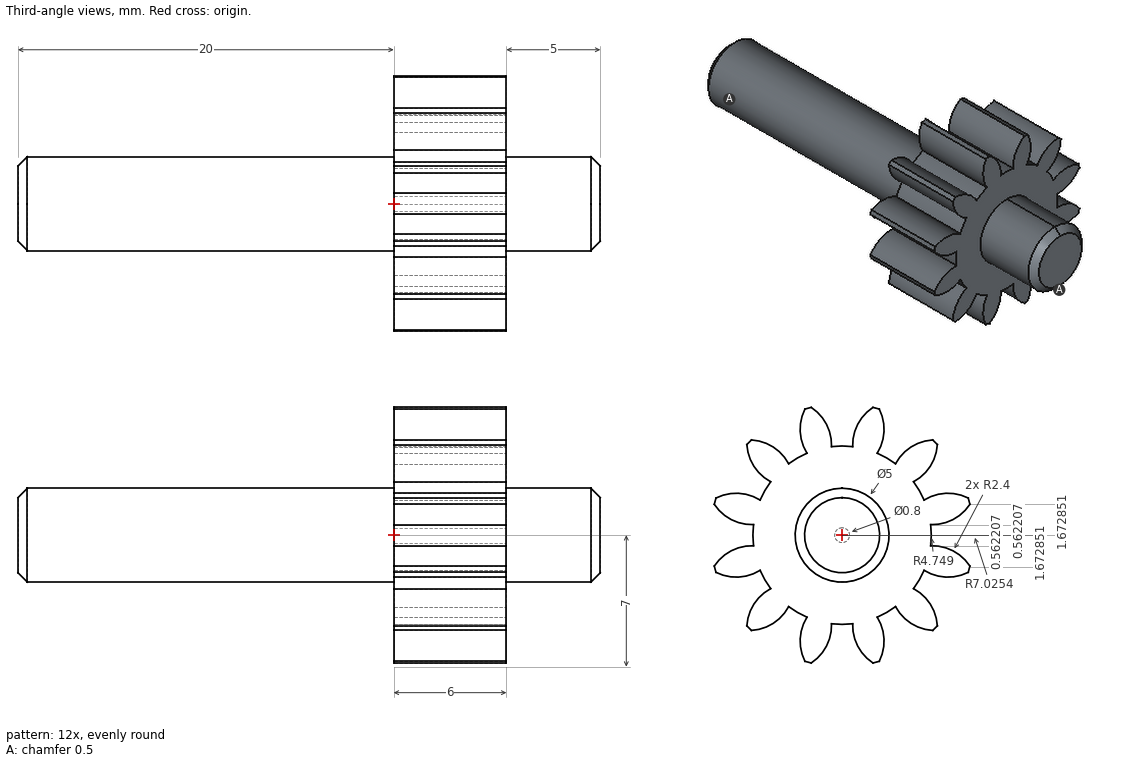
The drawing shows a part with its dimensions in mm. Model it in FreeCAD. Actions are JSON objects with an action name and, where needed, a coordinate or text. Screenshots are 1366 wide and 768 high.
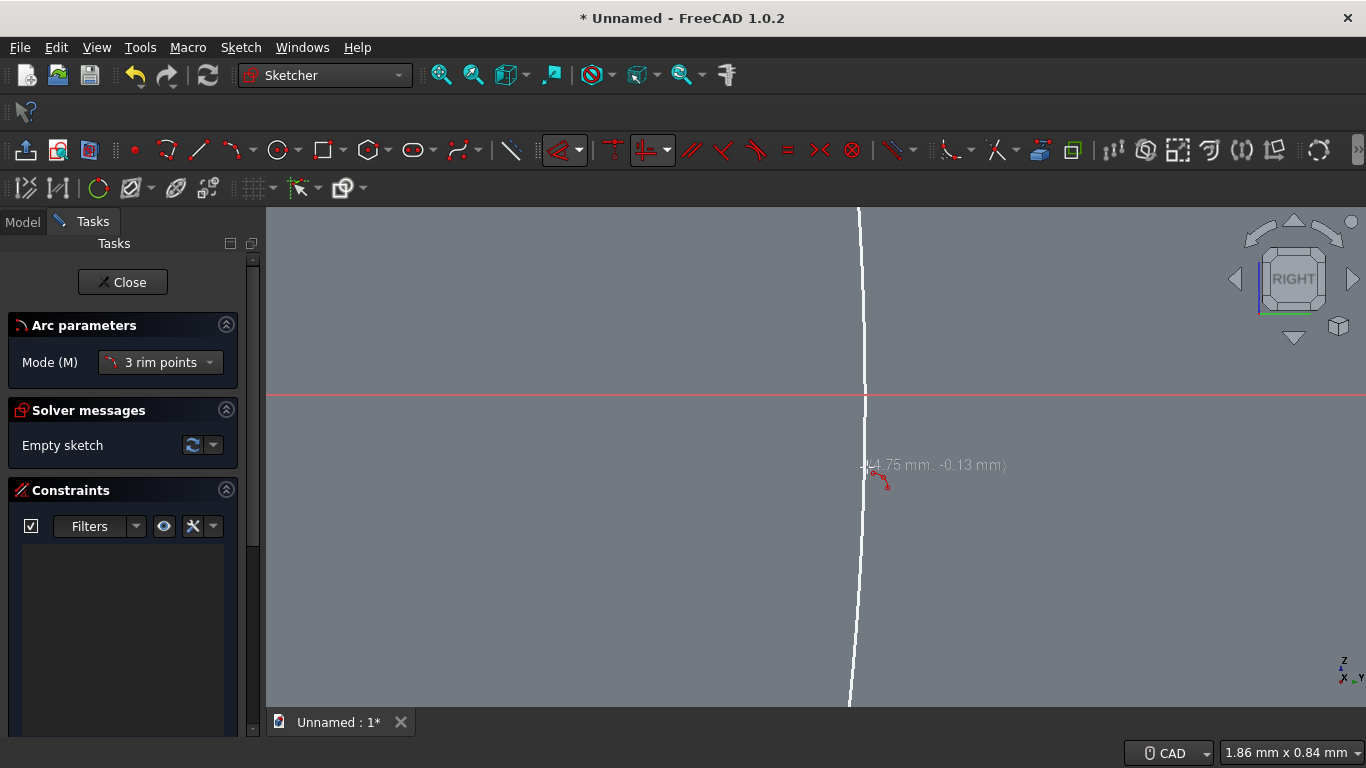
{"action": "left_click", "coordinate": [864, 461]}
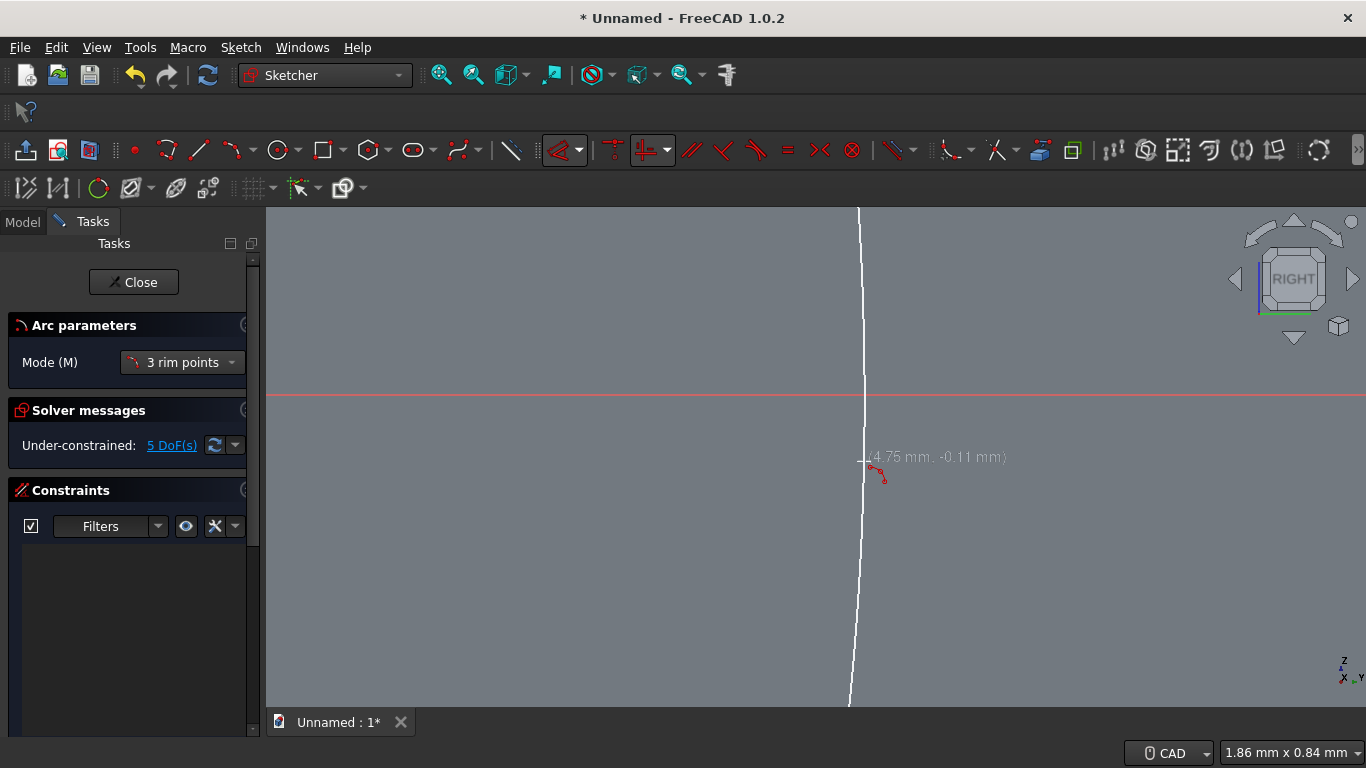
{"action": "scroll", "coordinate": [869, 469], "scroll_direction": "down", "scroll_amount": 9}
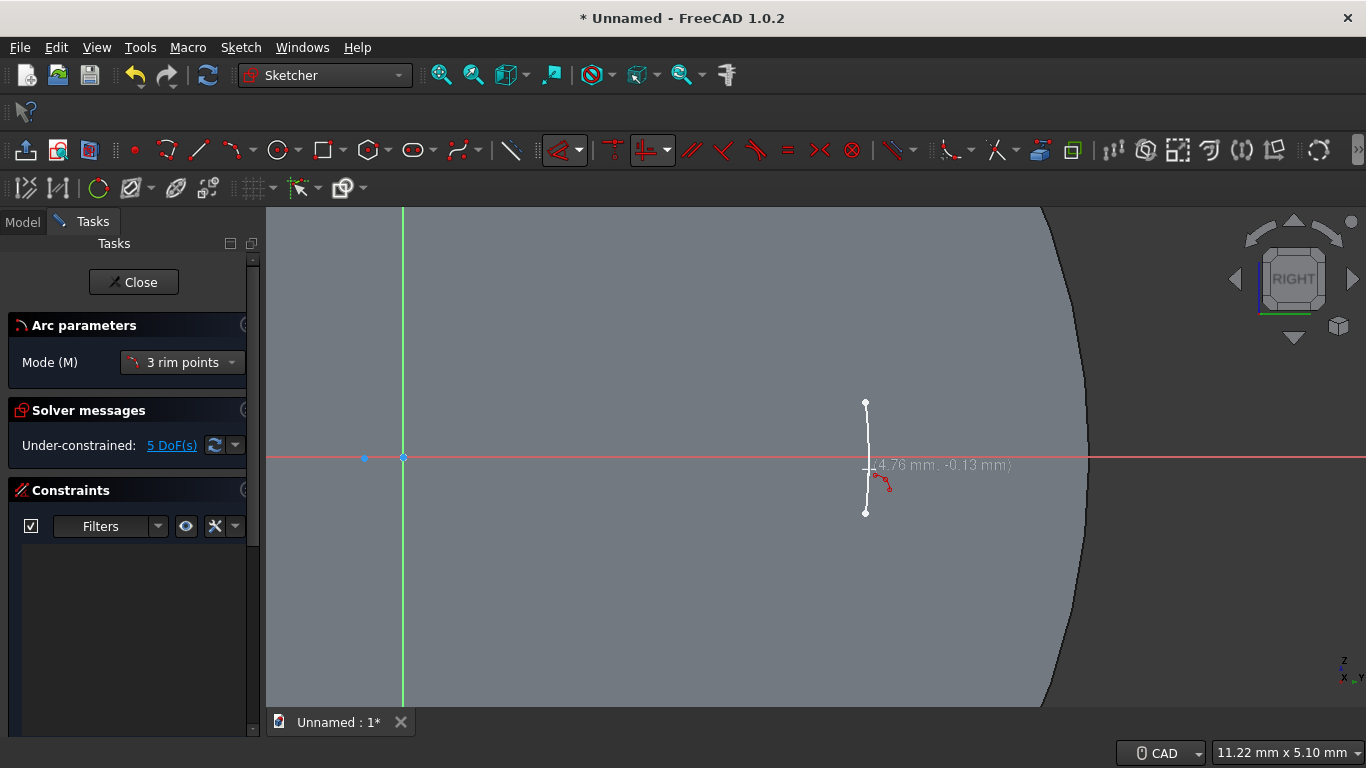
{"action": "left_click", "coordinate": [866, 514]}
{"action": "left_click", "coordinate": [1072, 621]}
{"action": "left_click", "coordinate": [983, 539]}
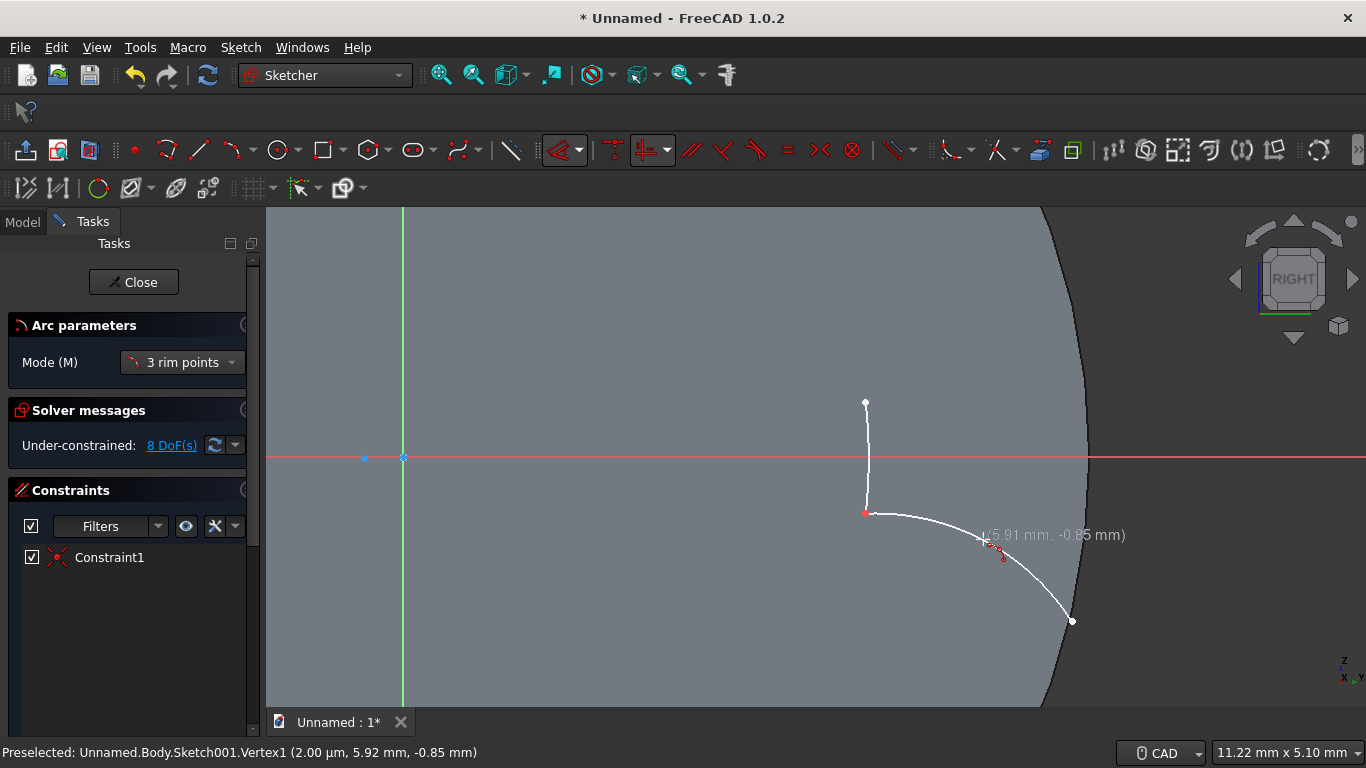
{"action": "left_click", "coordinate": [1072, 622]}
{"action": "left_click", "coordinate": [1072, 293]}
{"action": "left_click", "coordinate": [1091, 490]}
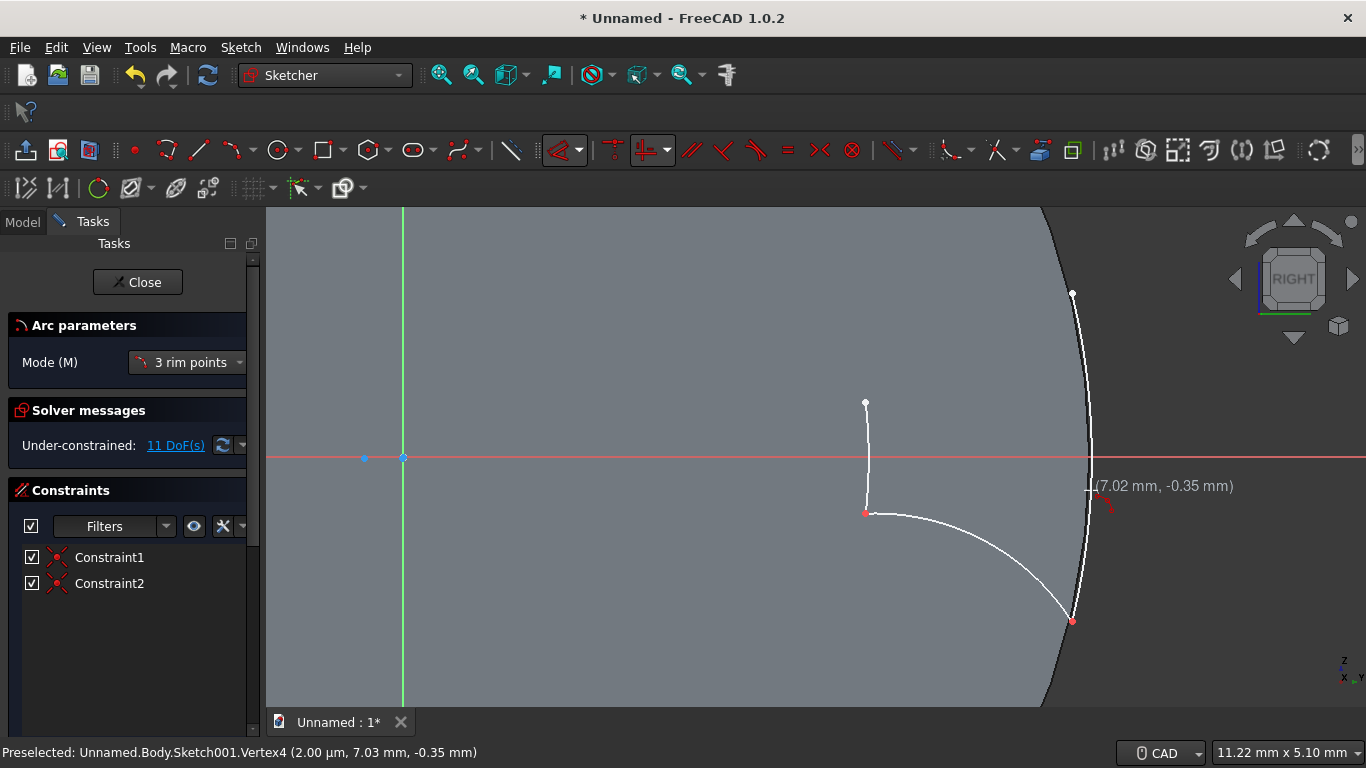
{"action": "left_click", "coordinate": [1072, 294]}
{"action": "left_click", "coordinate": [866, 403]}
{"action": "left_click", "coordinate": [983, 375]}
{"action": "key", "text": "Escape"}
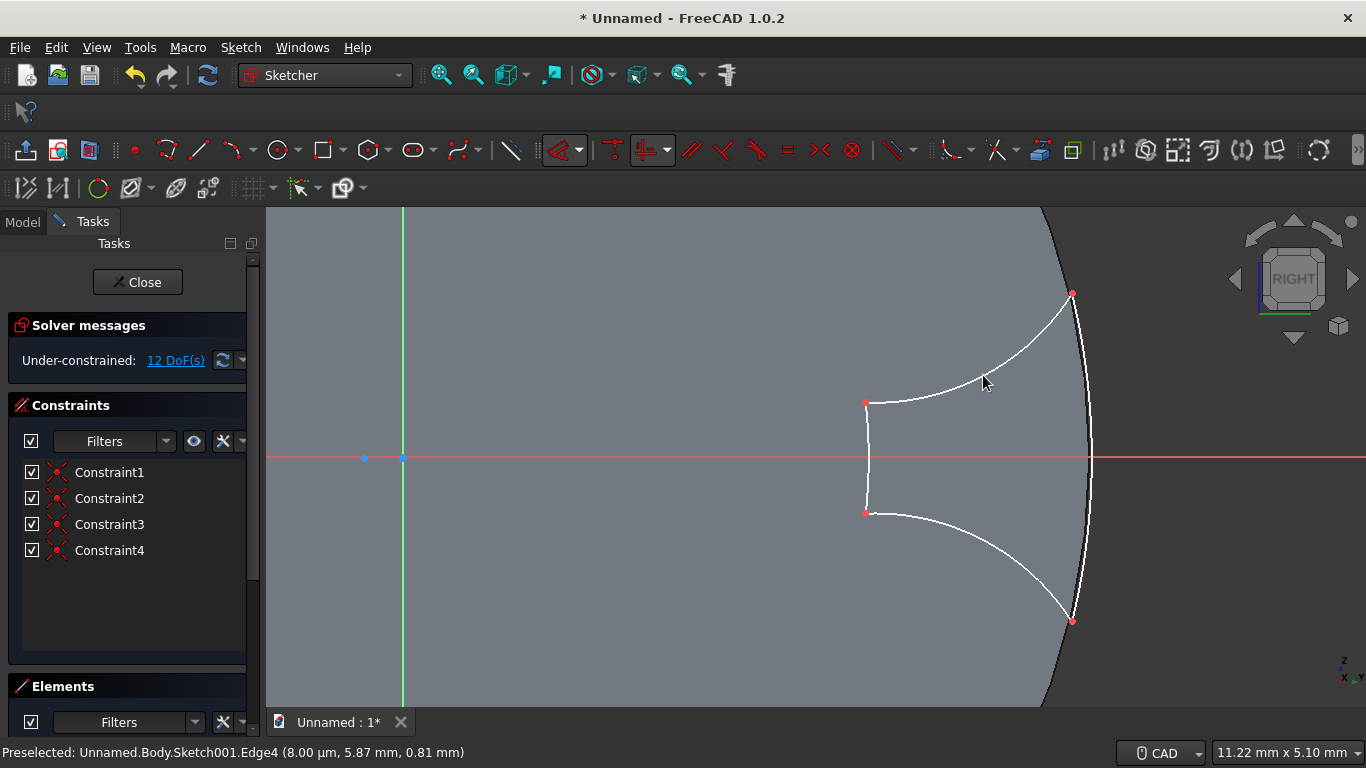
{"action": "left_click", "coordinate": [868, 480]}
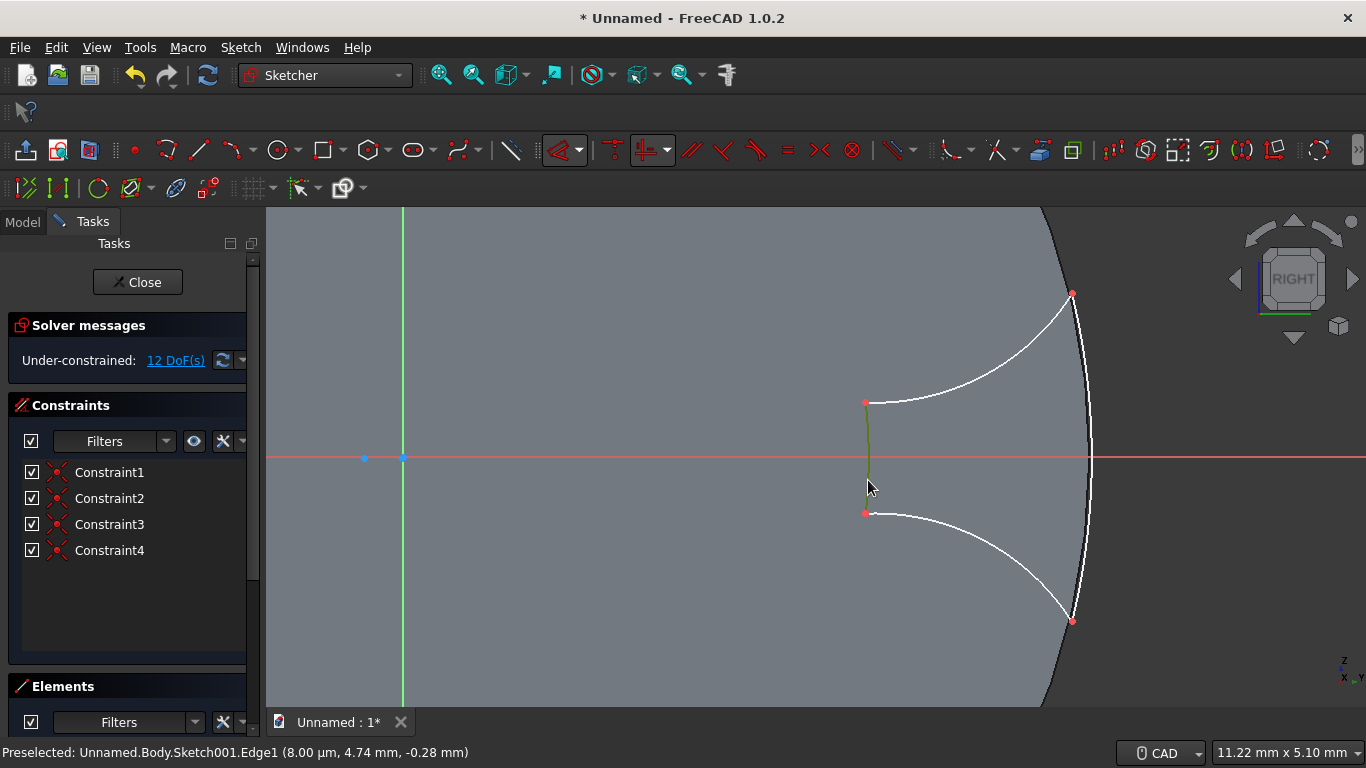
{"action": "left_click", "coordinate": [1089, 524]}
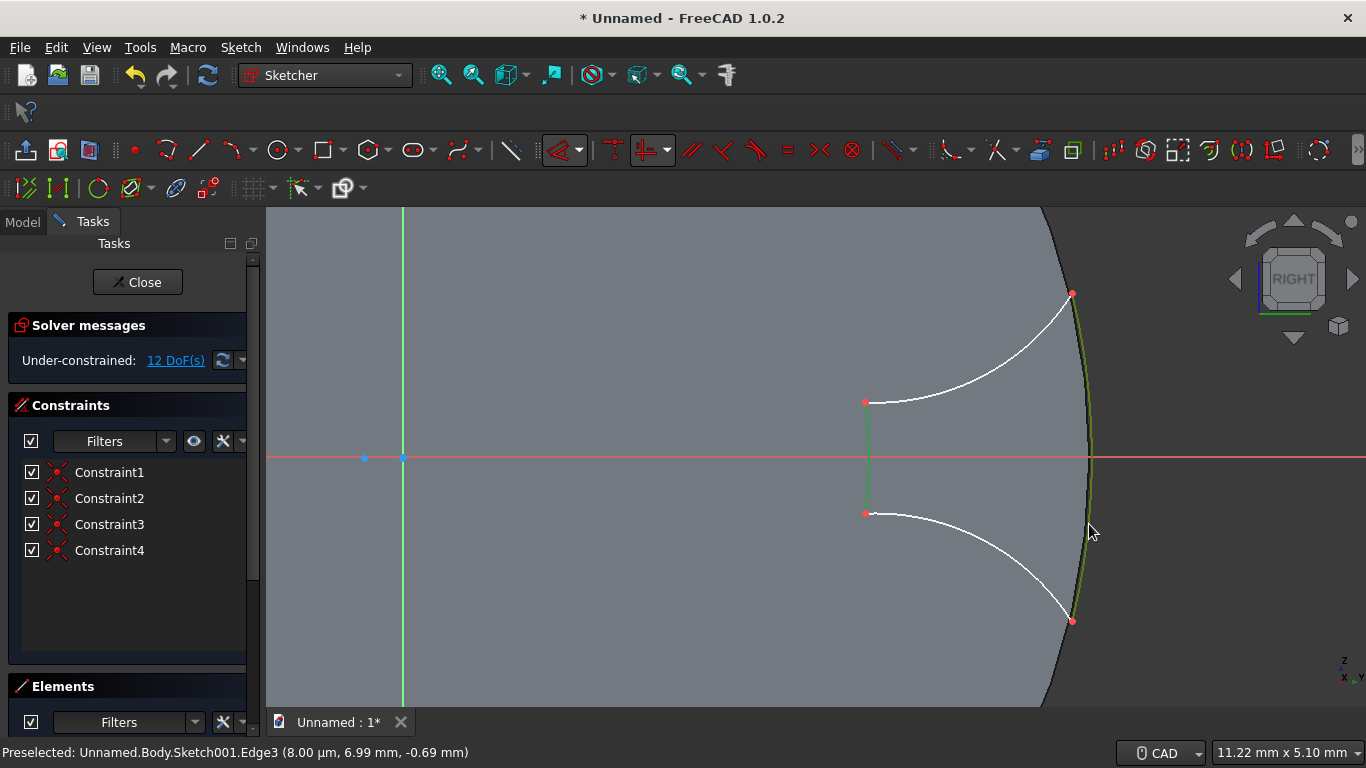
{"action": "key", "text": "c"}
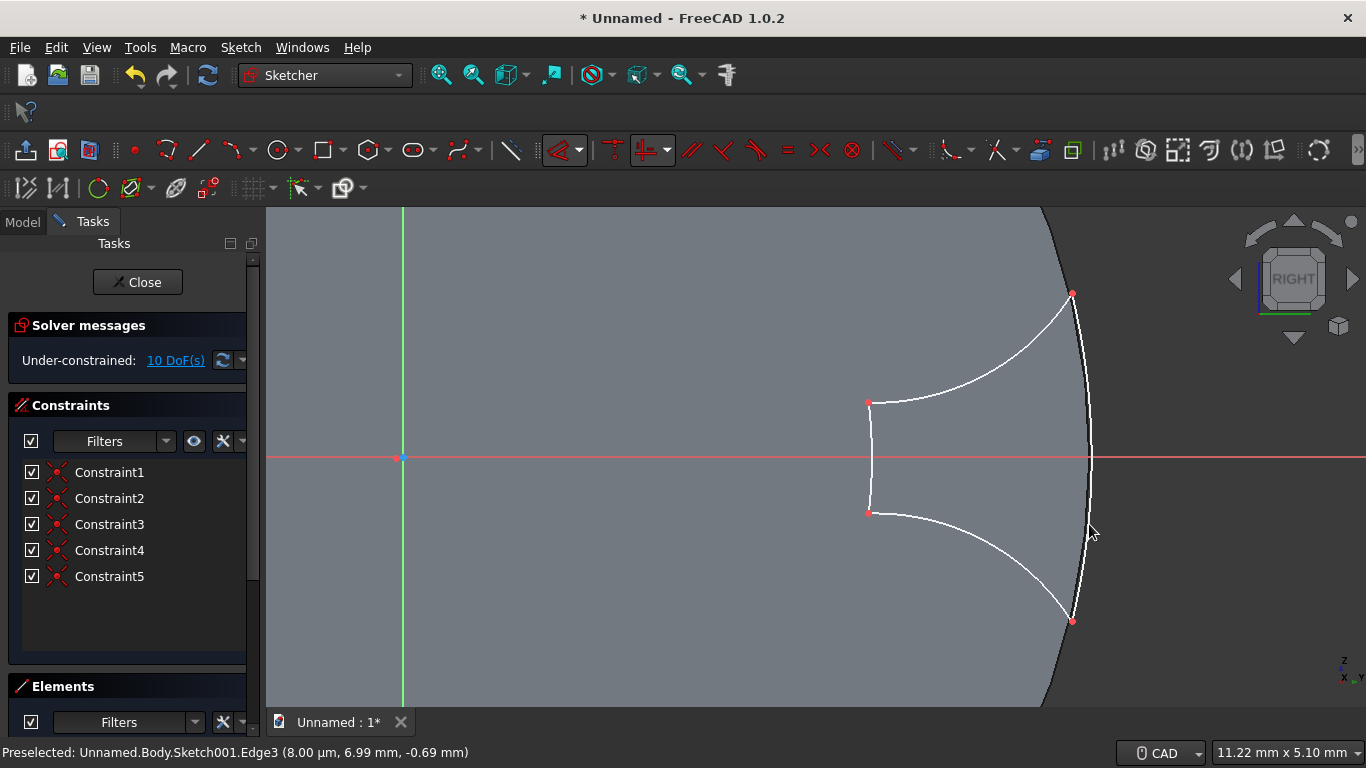
{"action": "left_click_drag", "start_coordinate": [386, 447], "coordinate": [413, 468]}